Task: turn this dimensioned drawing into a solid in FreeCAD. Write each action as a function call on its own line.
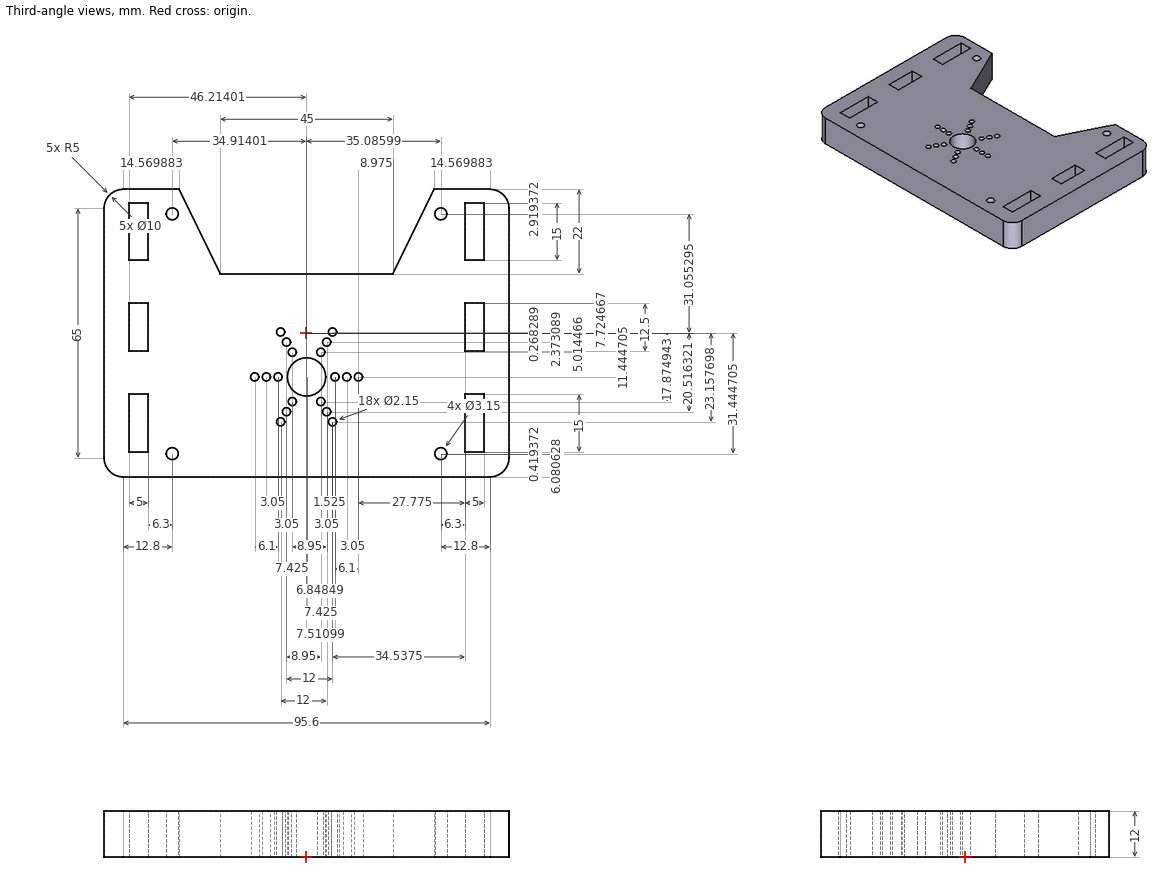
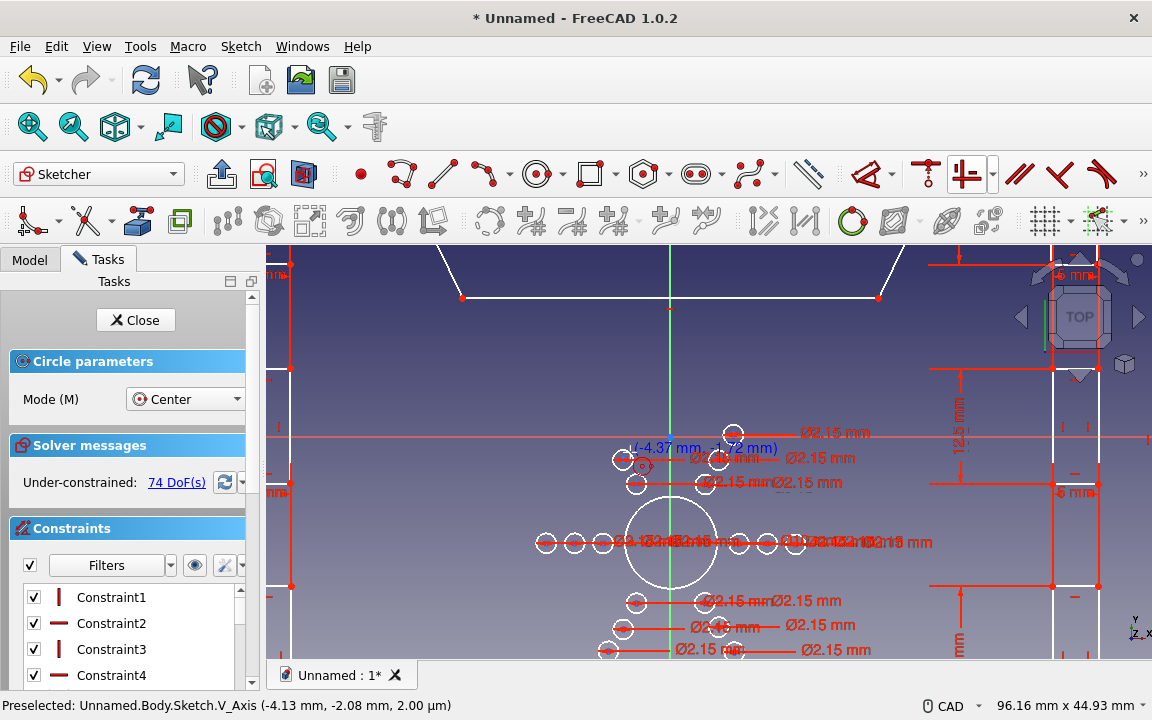
scroll(609, 435, up, 10)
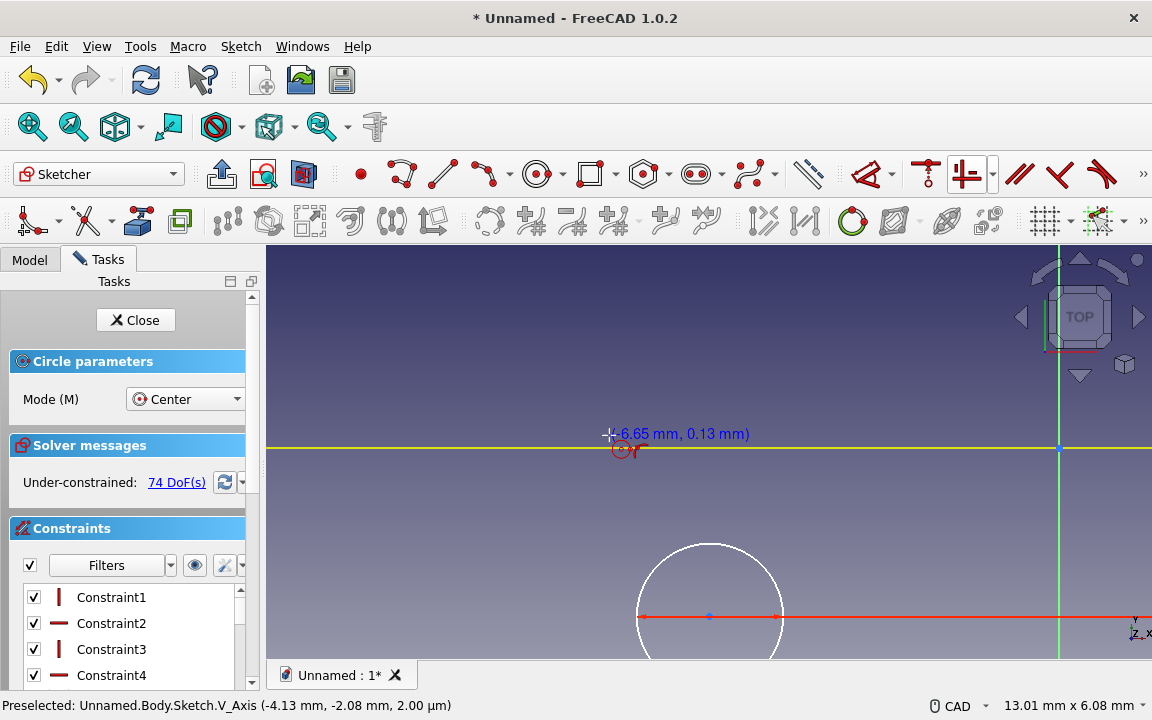
click(605, 430)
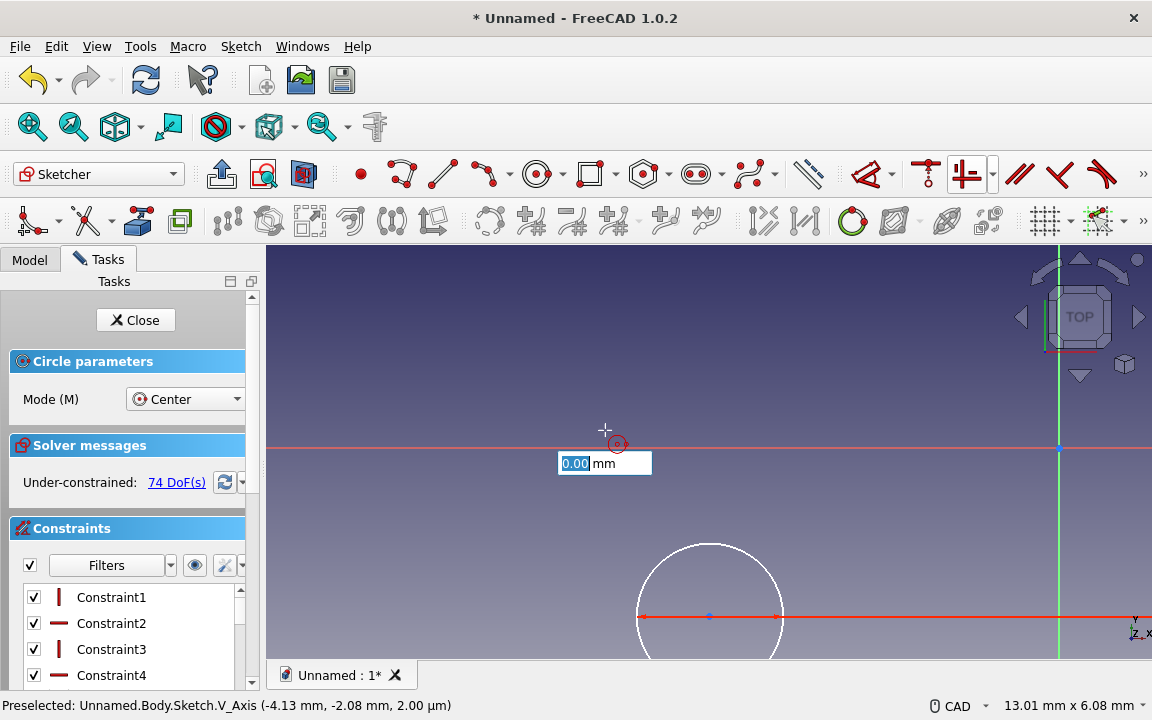
scroll(618, 452, down, 15)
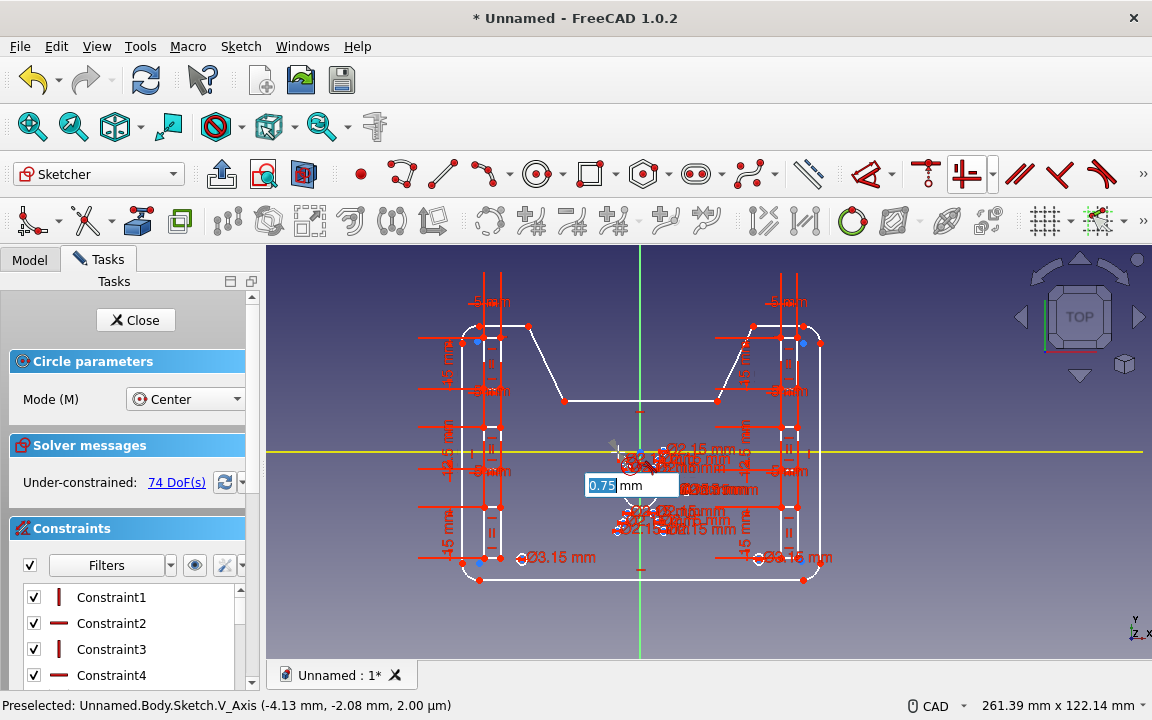
scroll(620, 449, up, 8)
move(620, 446)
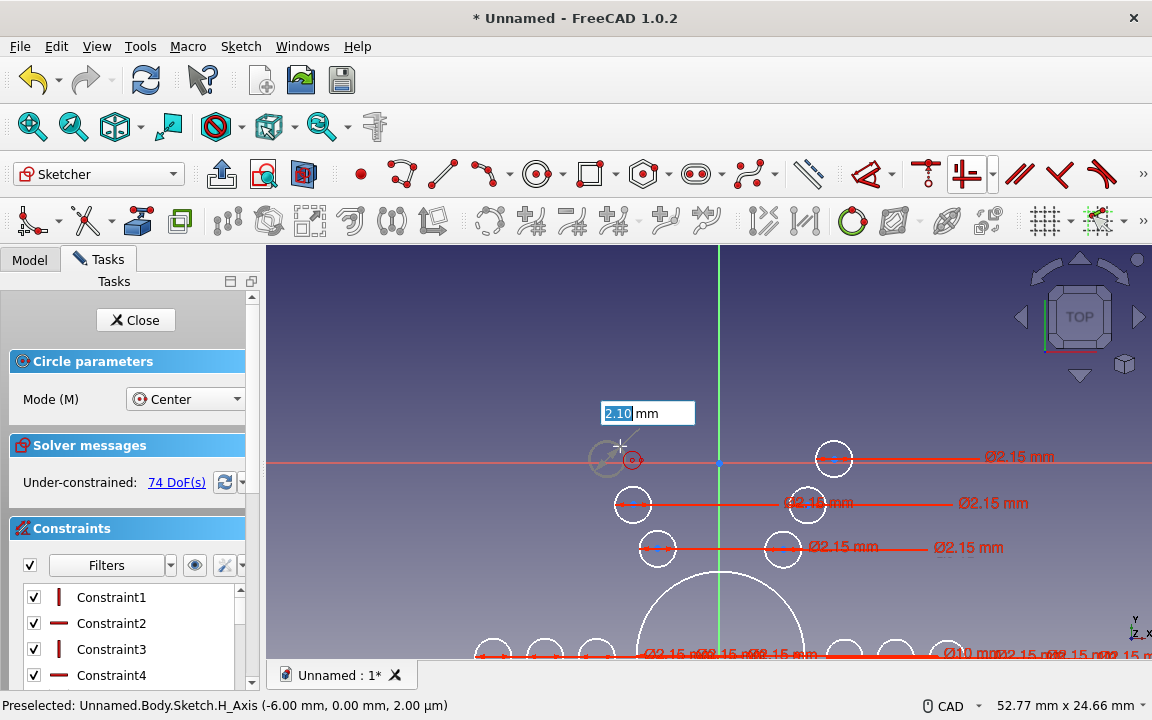
text(2.15)
key(Return)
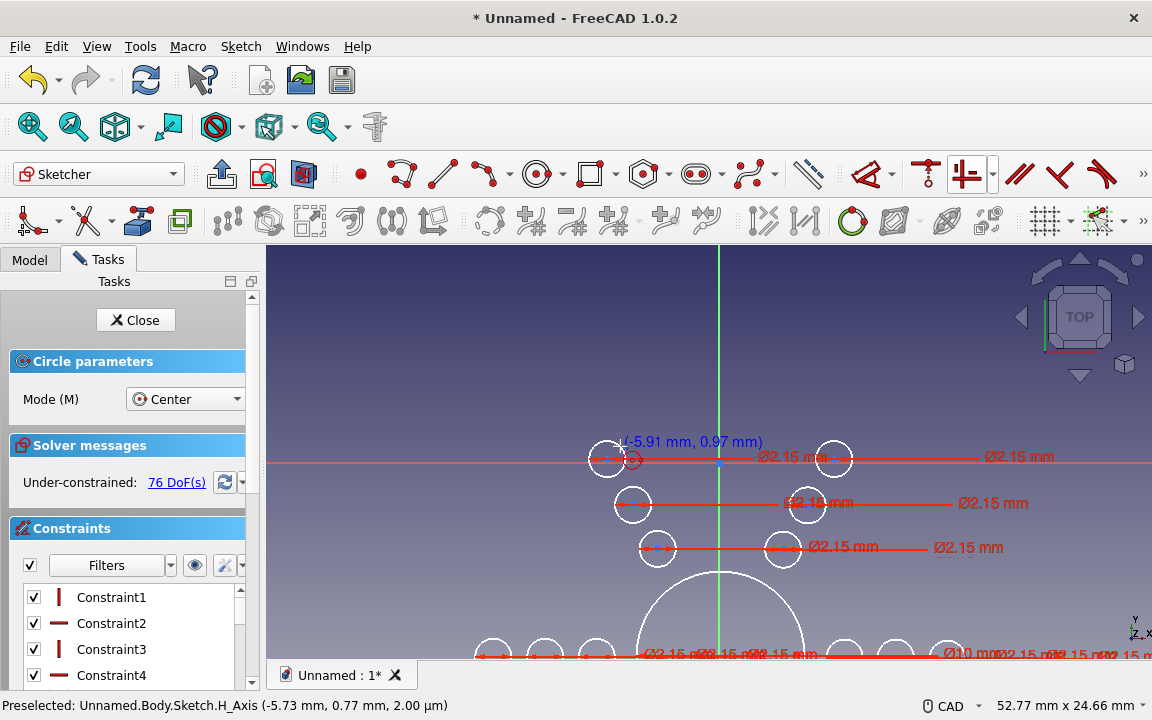
scroll(620, 449, down, 8)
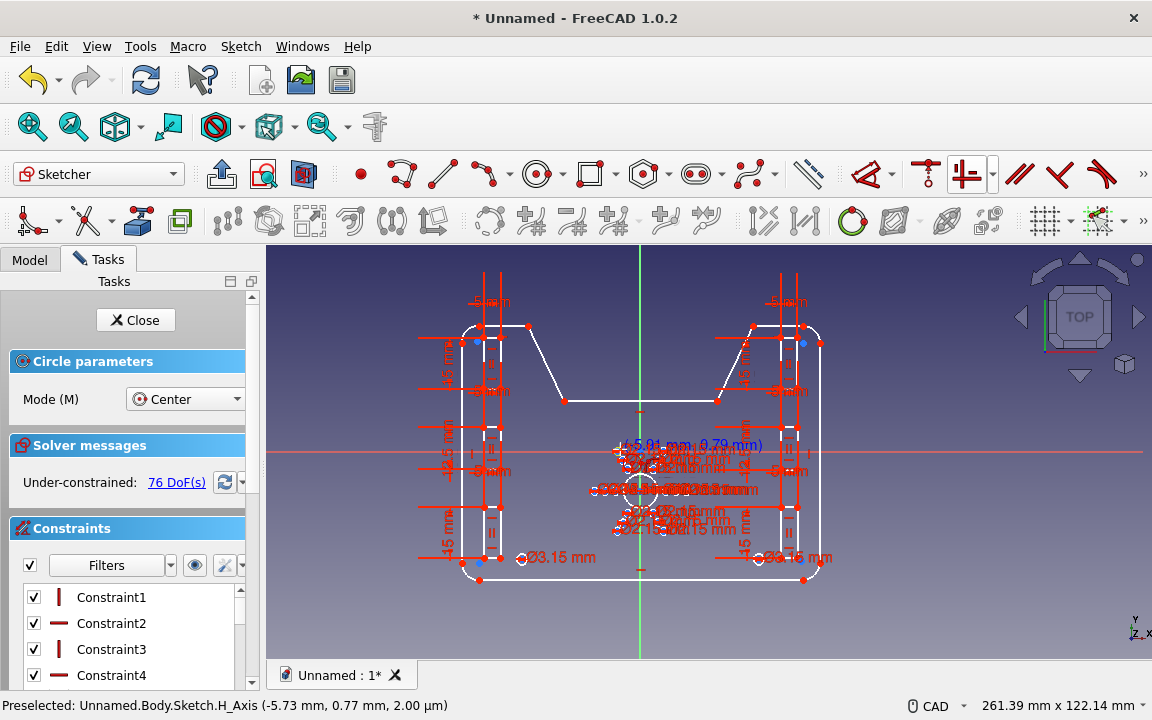
scroll(759, 347, up, 8)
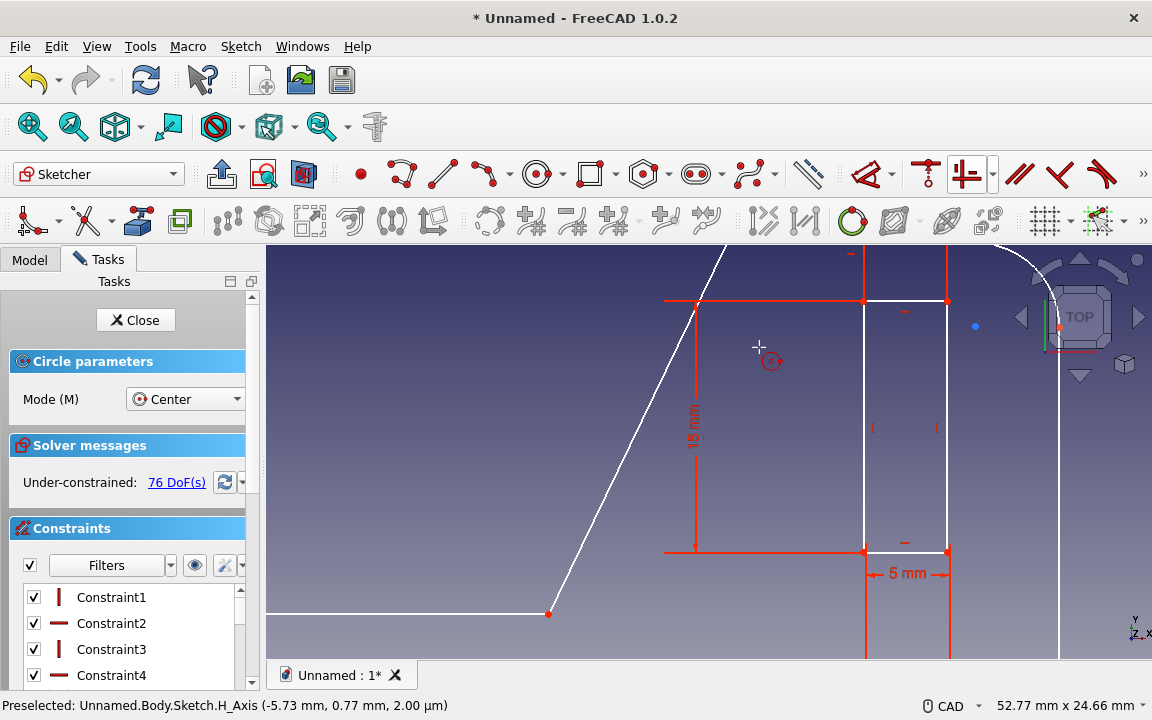
scroll(759, 347, down, 8)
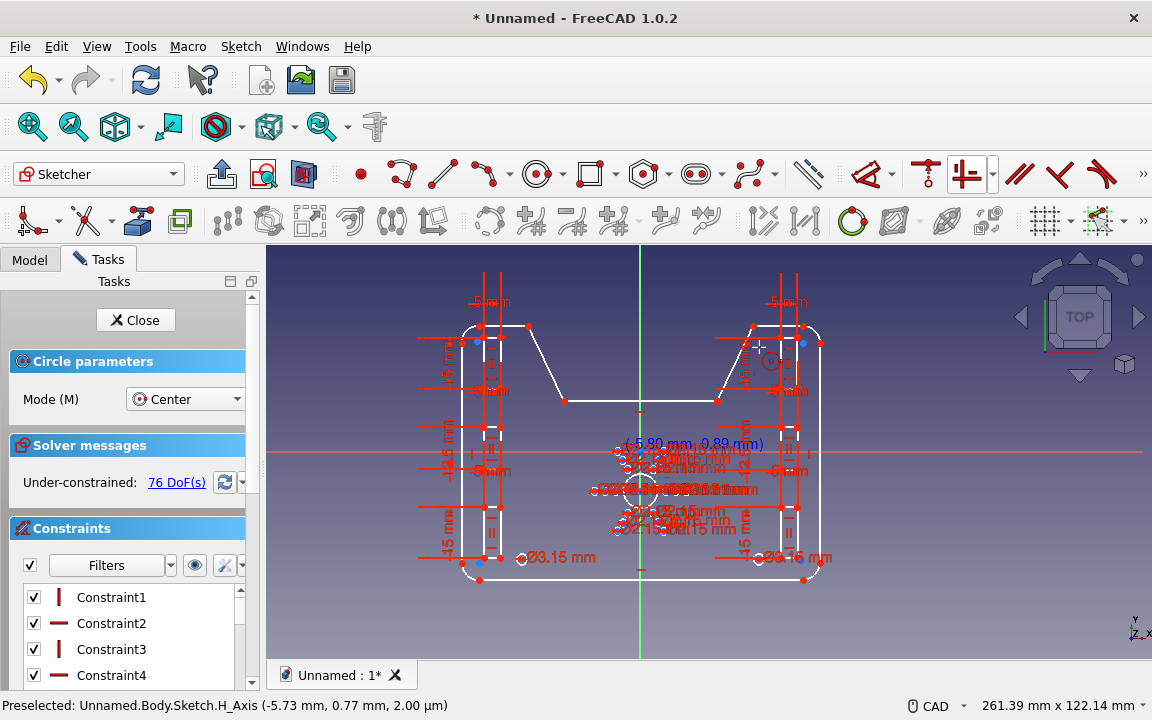
click(759, 347)
move(763, 343)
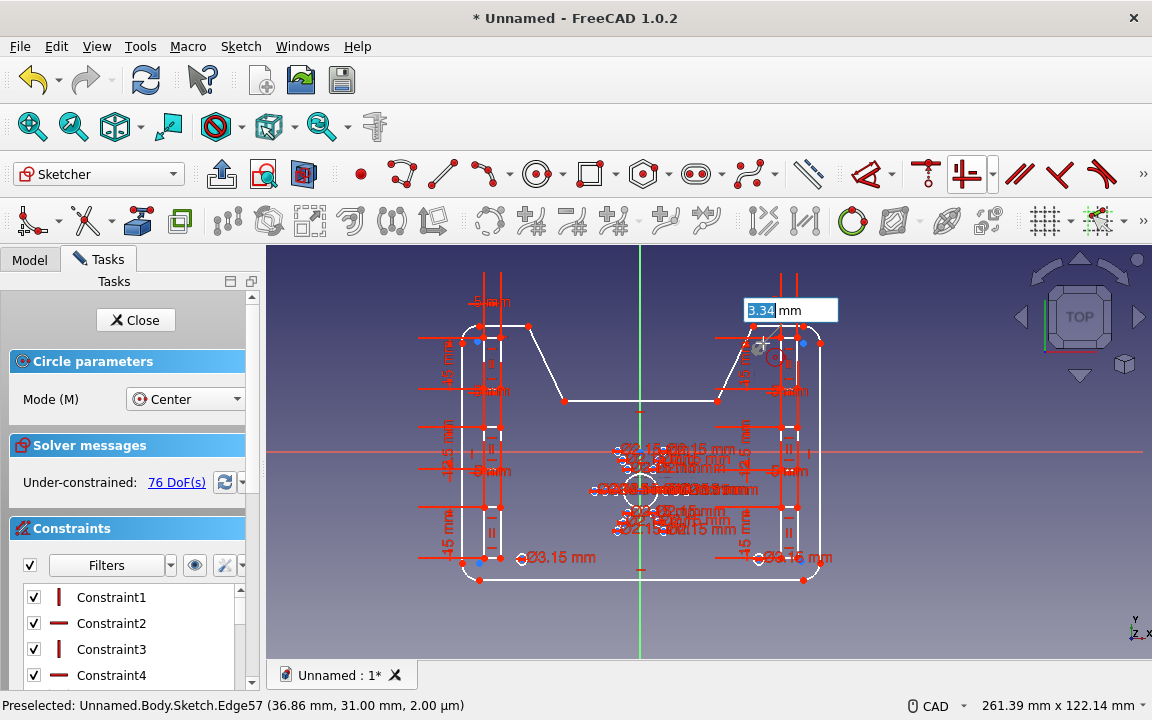
text(3.15)
key(Return)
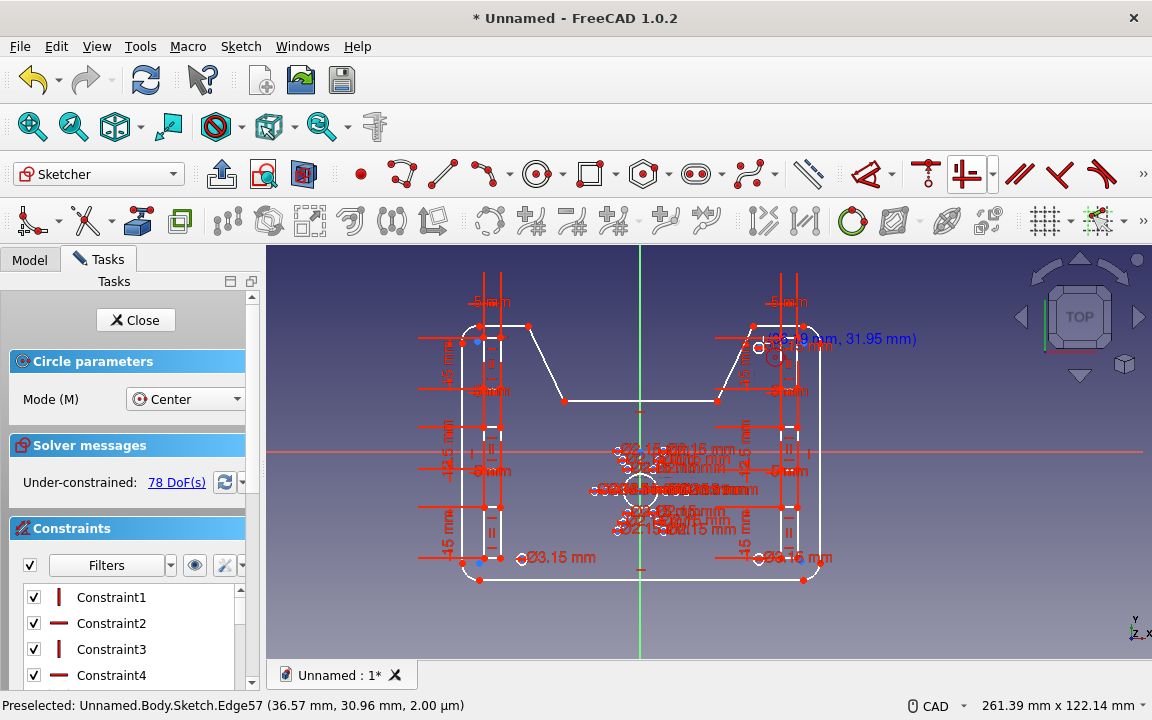
scroll(522, 347, up, 8)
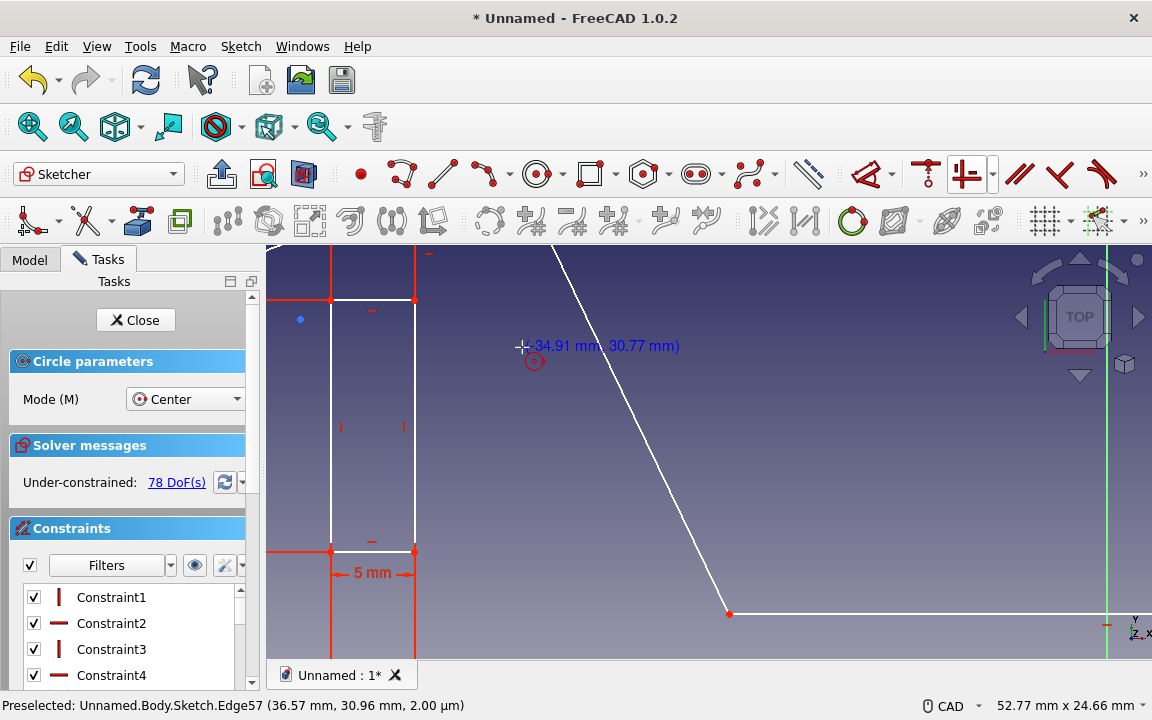
scroll(522, 347, down, 8)